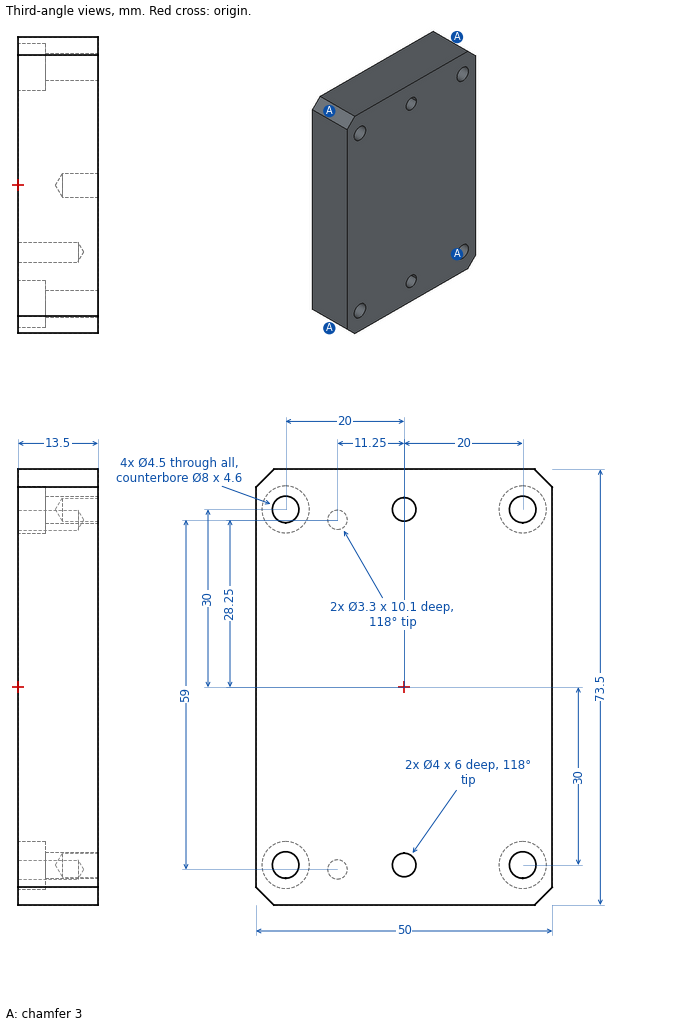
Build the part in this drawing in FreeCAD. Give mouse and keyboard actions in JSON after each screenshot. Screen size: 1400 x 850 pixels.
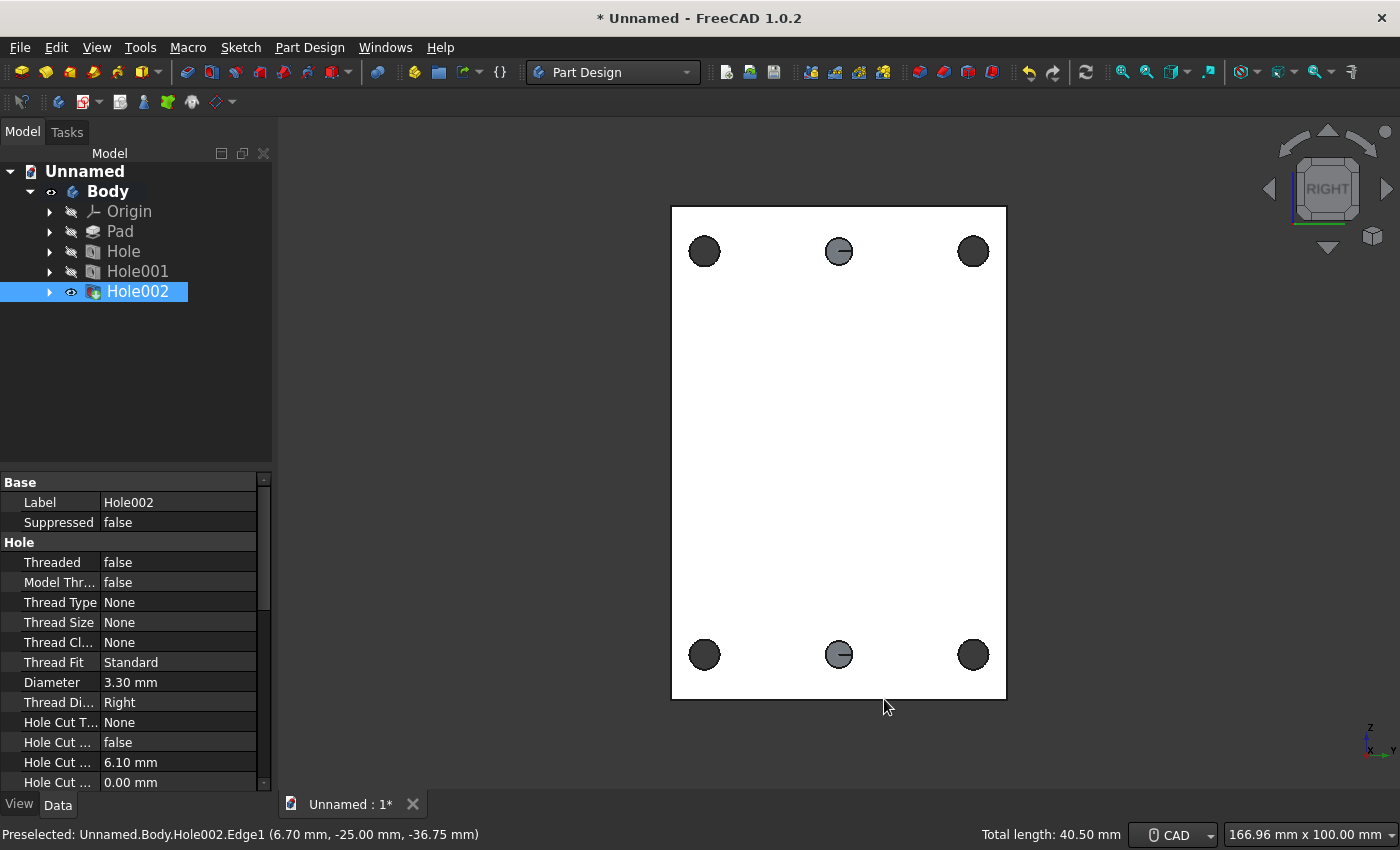
{"action": "key", "text": "5"}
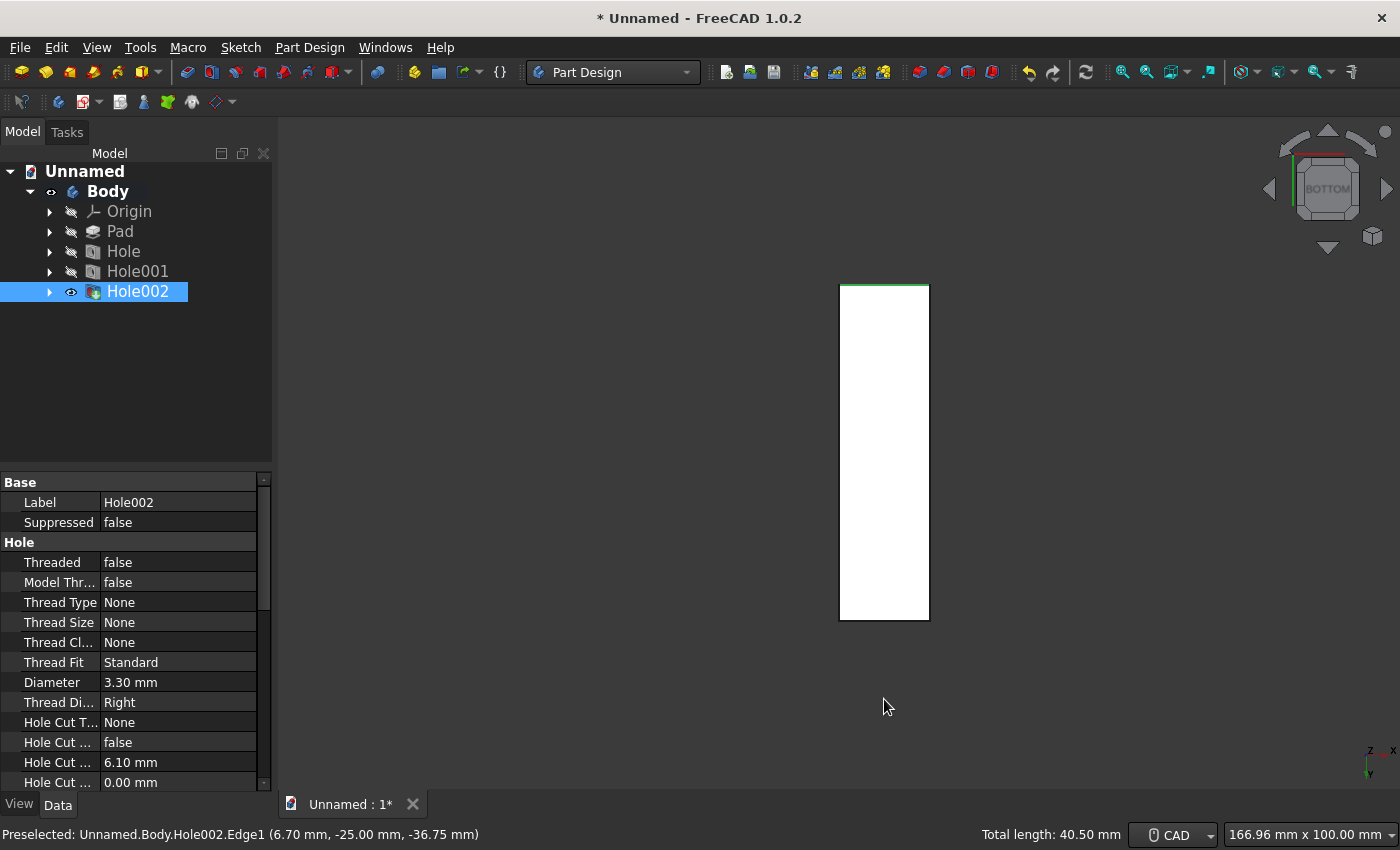
{"action": "left_click", "coordinate": [884, 620], "text": "ctrl"}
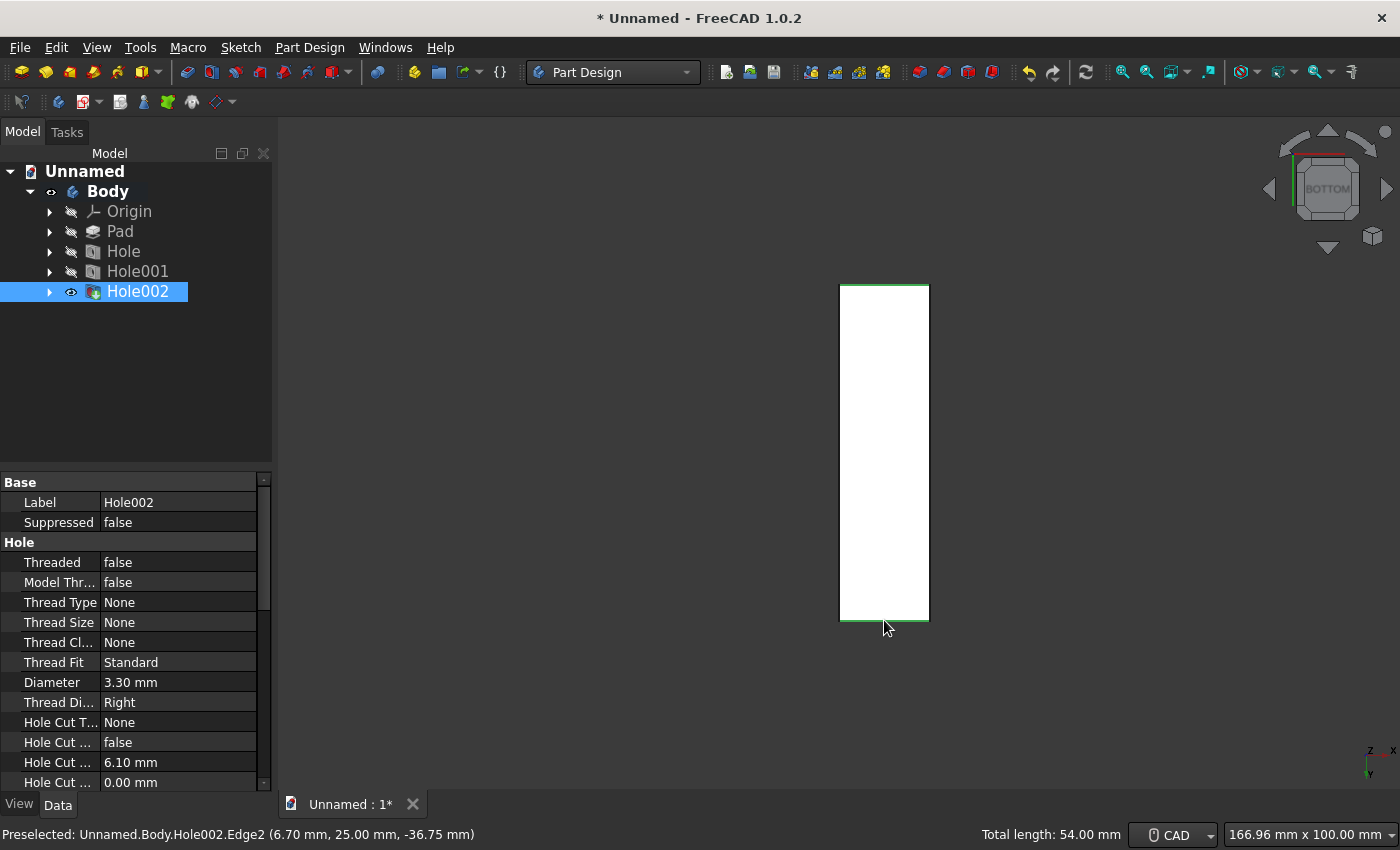
{"action": "left_click", "coordinate": [944, 72]}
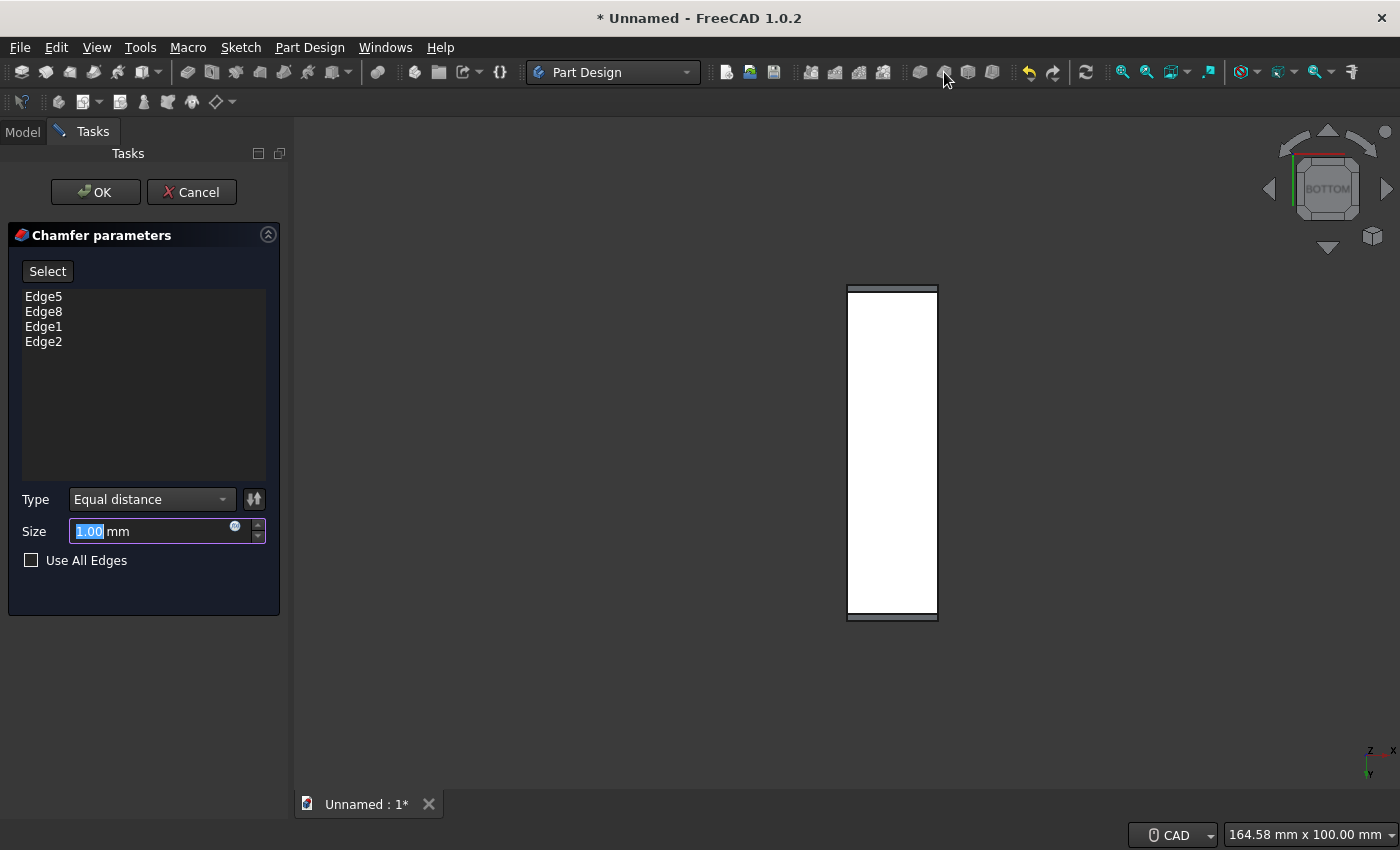
{"action": "type", "text": "3"}
{"action": "key", "text": "Tab"}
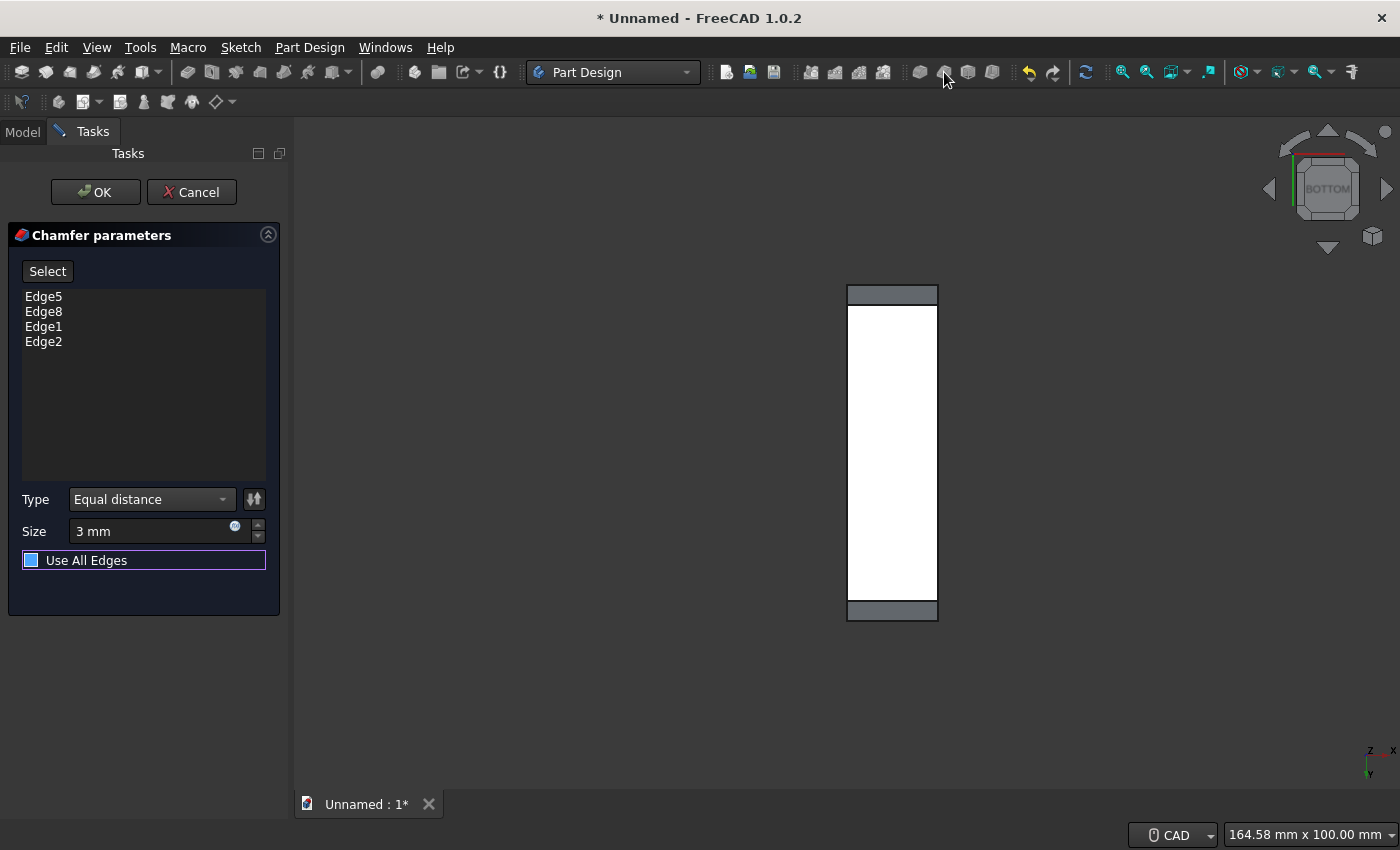
{"action": "left_click", "coordinate": [96, 192]}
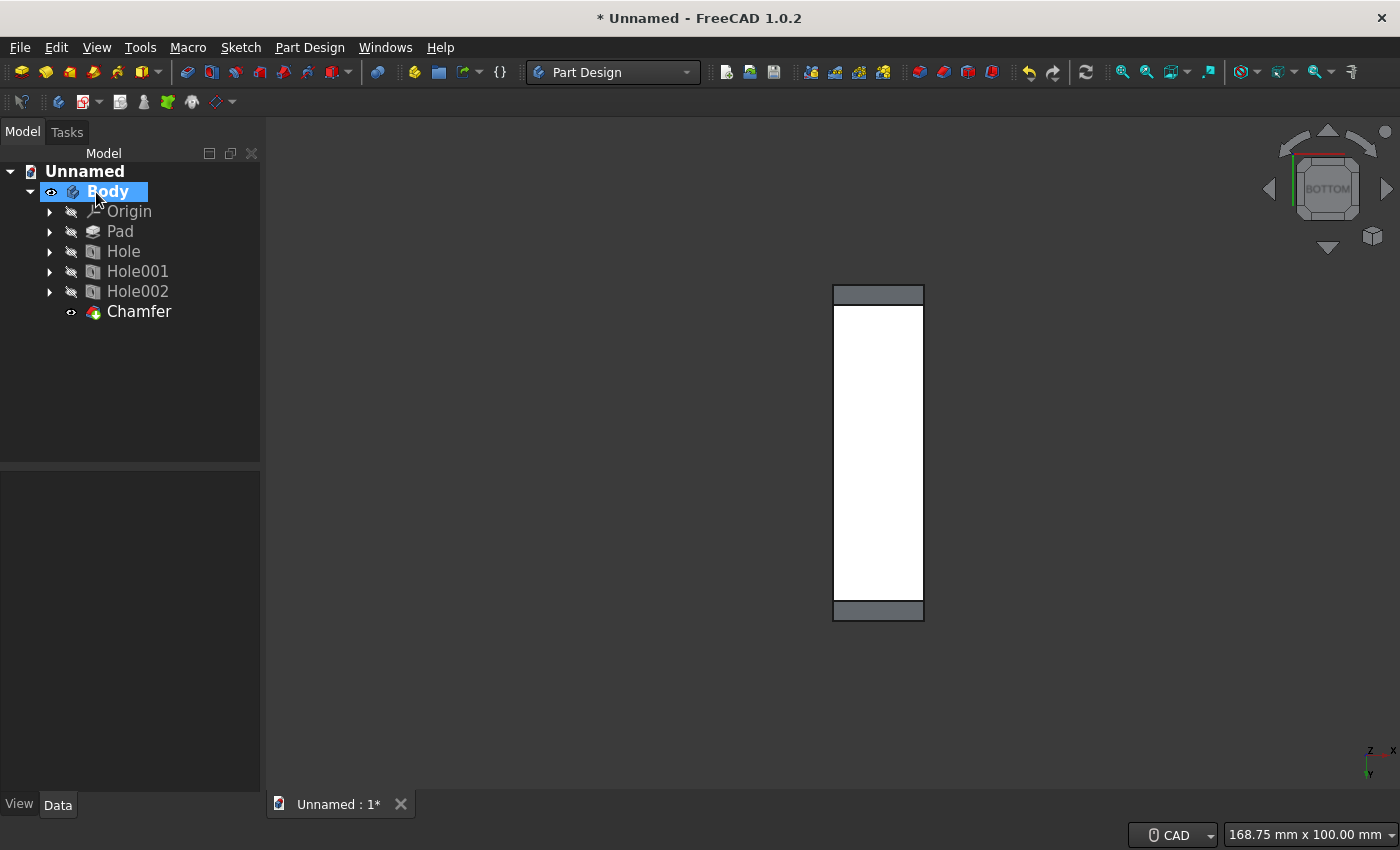
{"action": "key", "text": "0"}